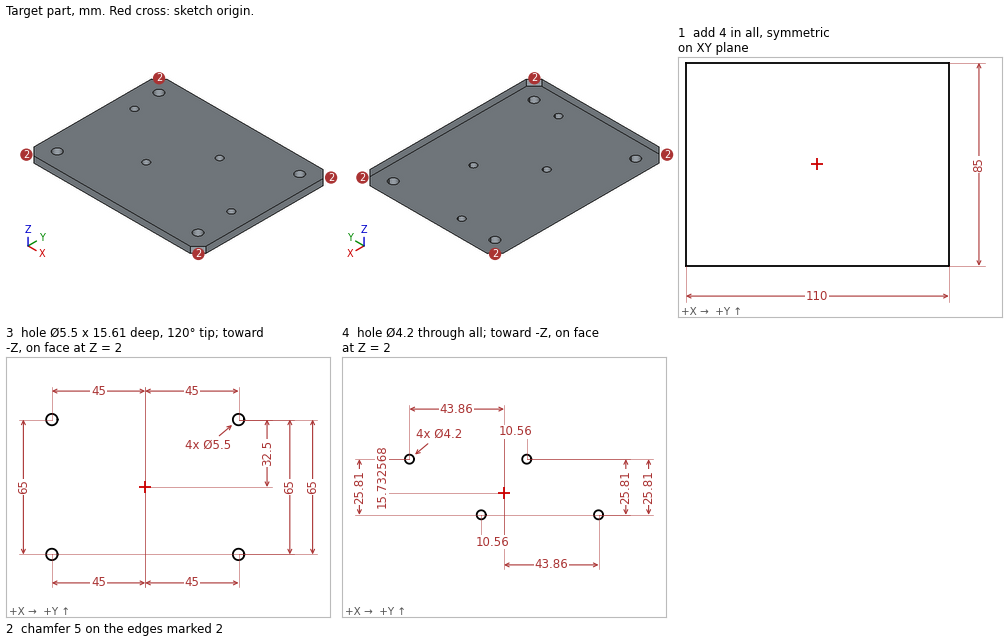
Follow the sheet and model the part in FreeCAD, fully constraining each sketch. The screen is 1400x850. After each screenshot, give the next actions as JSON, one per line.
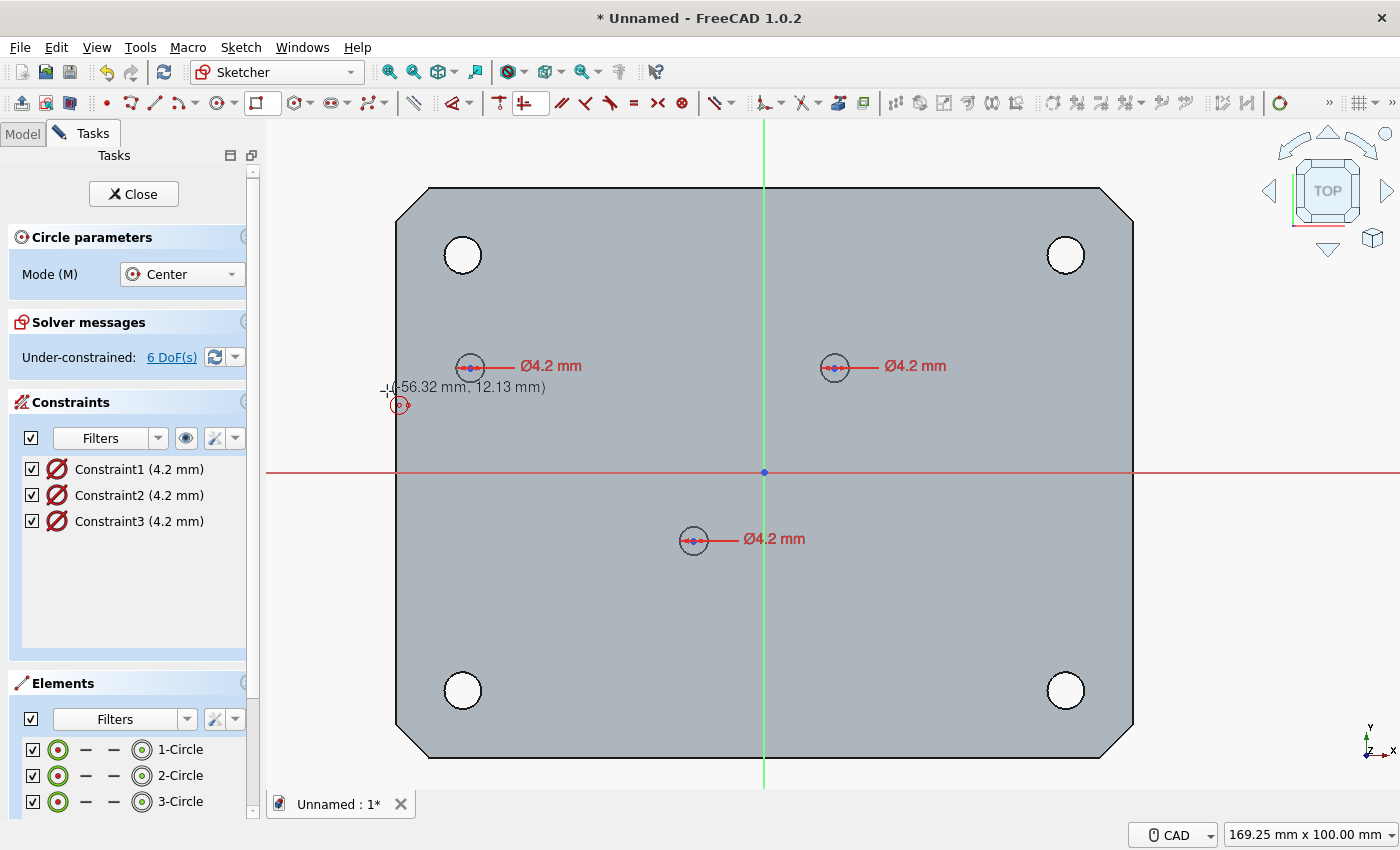
{"action": "scroll", "coordinate": [1058, 540], "scroll_direction": "up", "scroll_amount": 3}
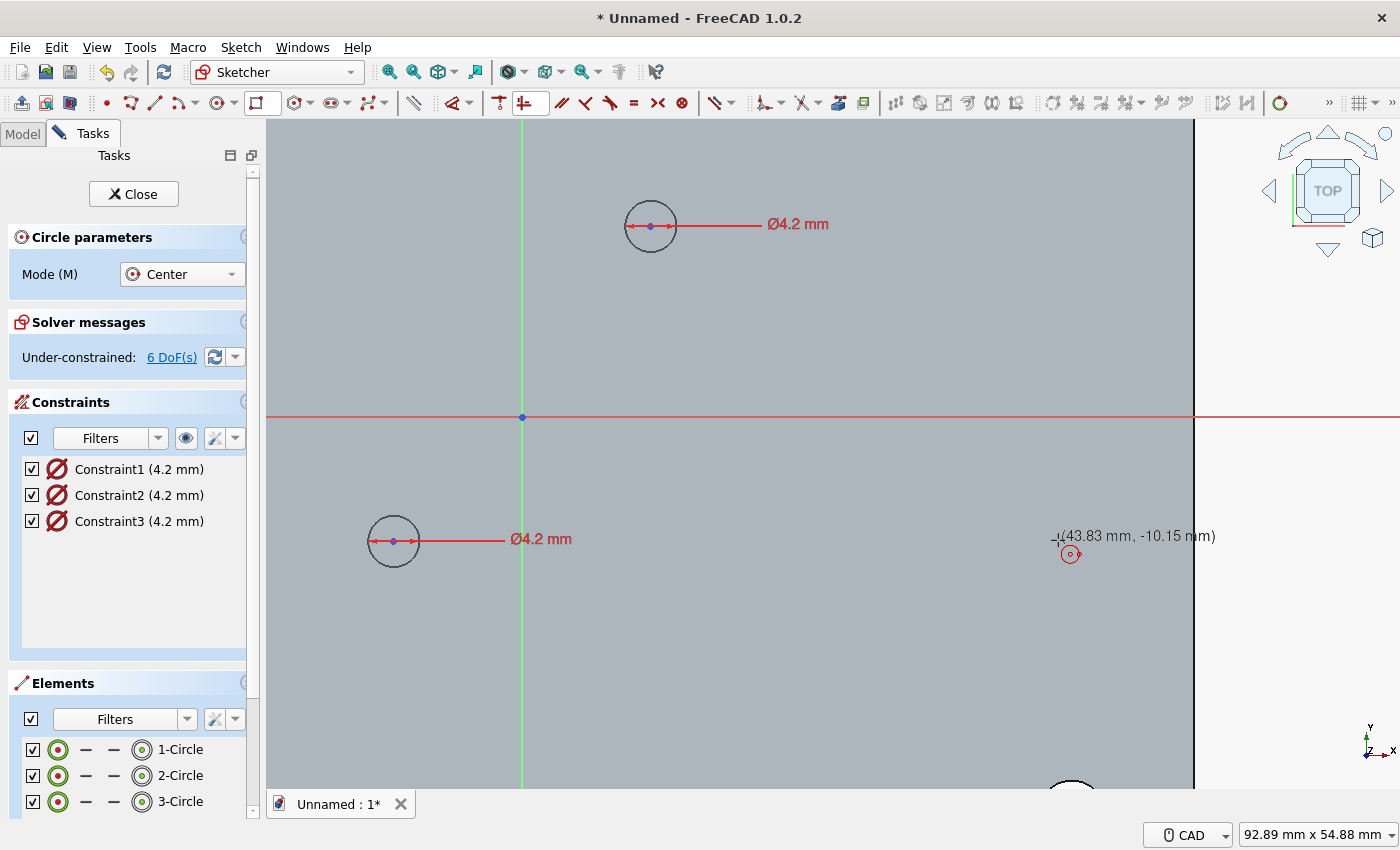
{"action": "left_click", "coordinate": [1058, 540]}
{"action": "mouse_move", "coordinate": [1076, 522]}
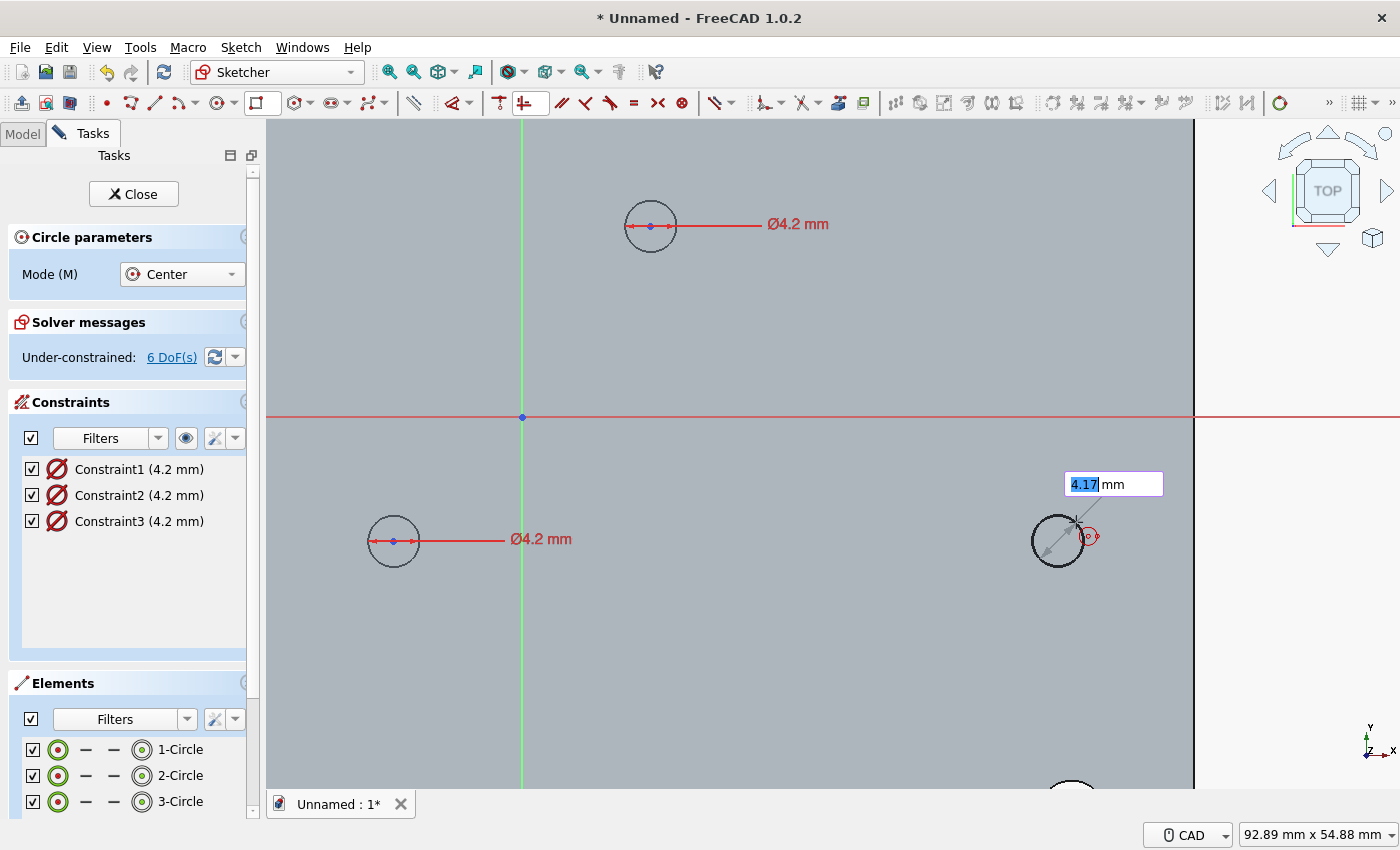
{"action": "type", "text": "4.2"}
{"action": "key", "text": "Return"}
{"action": "key", "text": "Escape"}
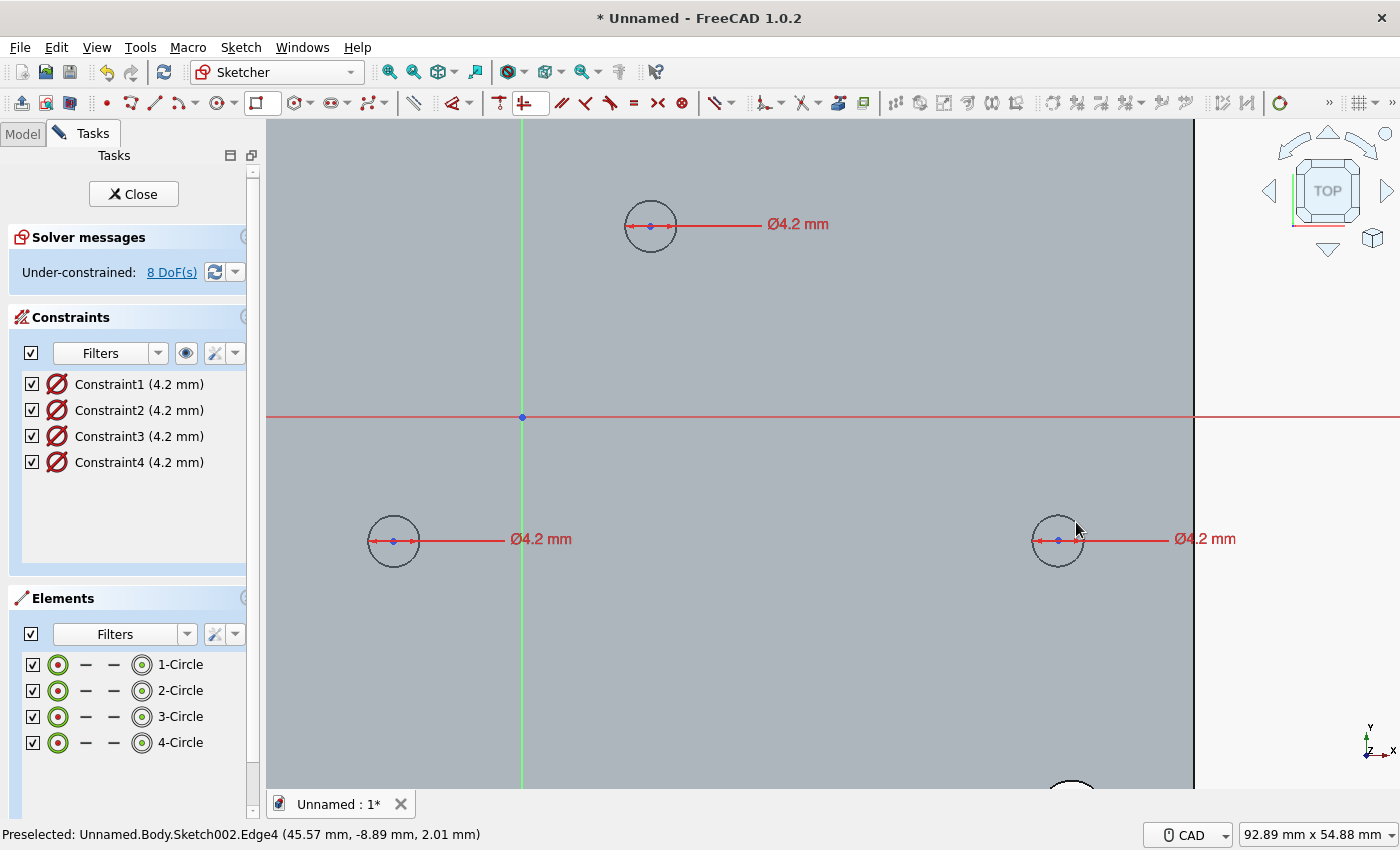
{"action": "key", "text": "d"}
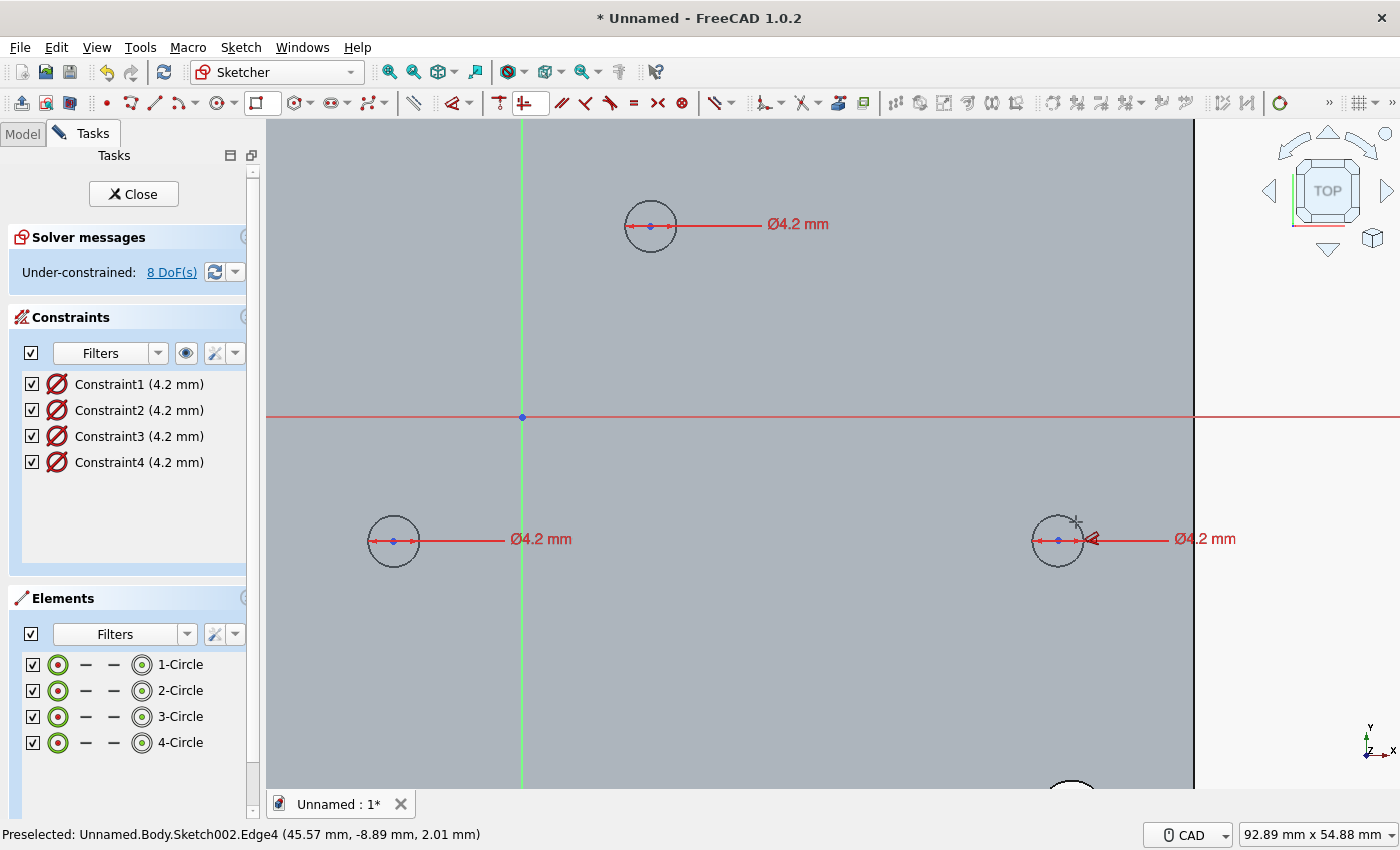
{"action": "scroll", "coordinate": [1059, 541], "scroll_direction": "down", "scroll_amount": 3}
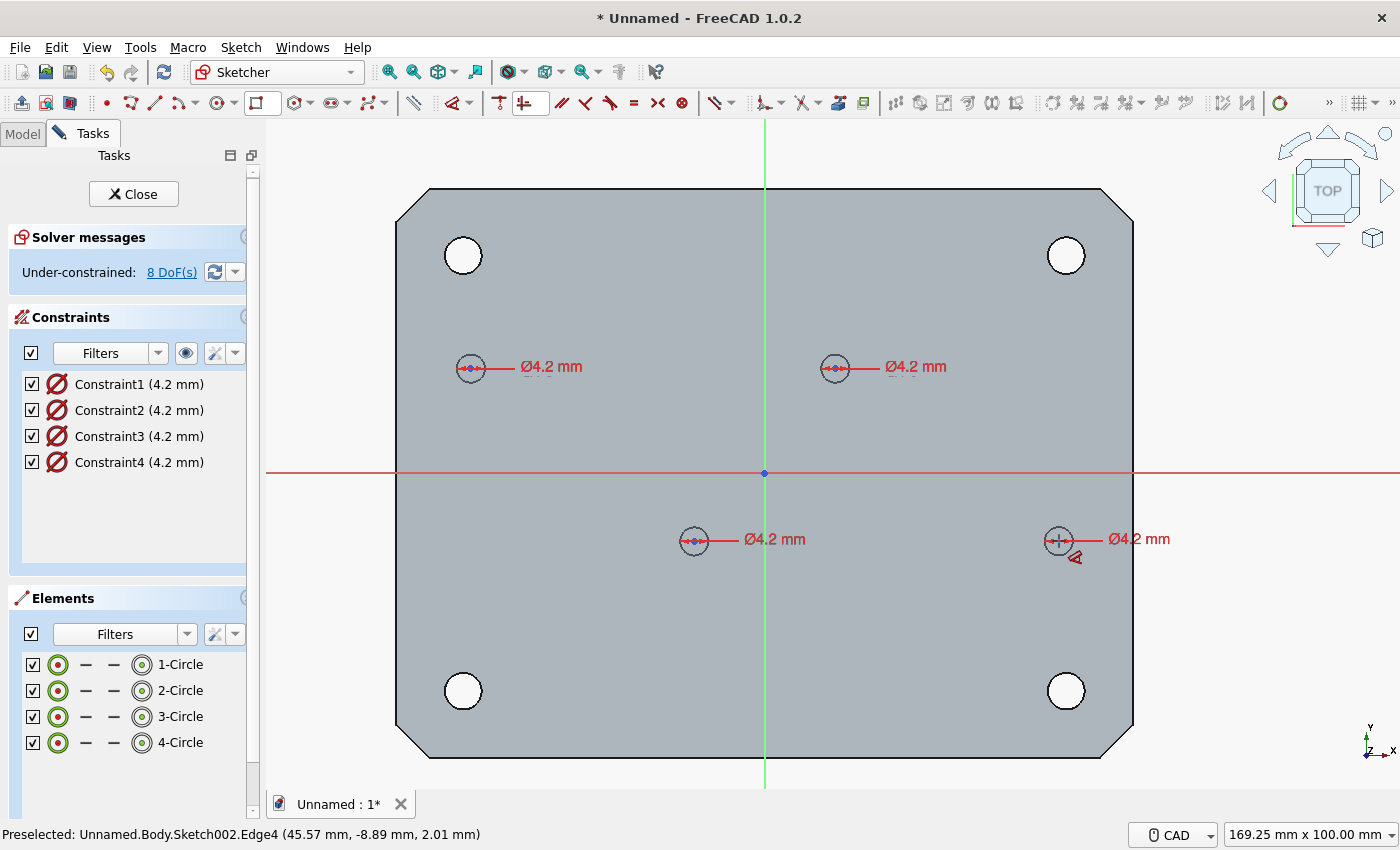
{"action": "left_click", "coordinate": [471, 369]}
{"action": "left_click", "coordinate": [618, 335]}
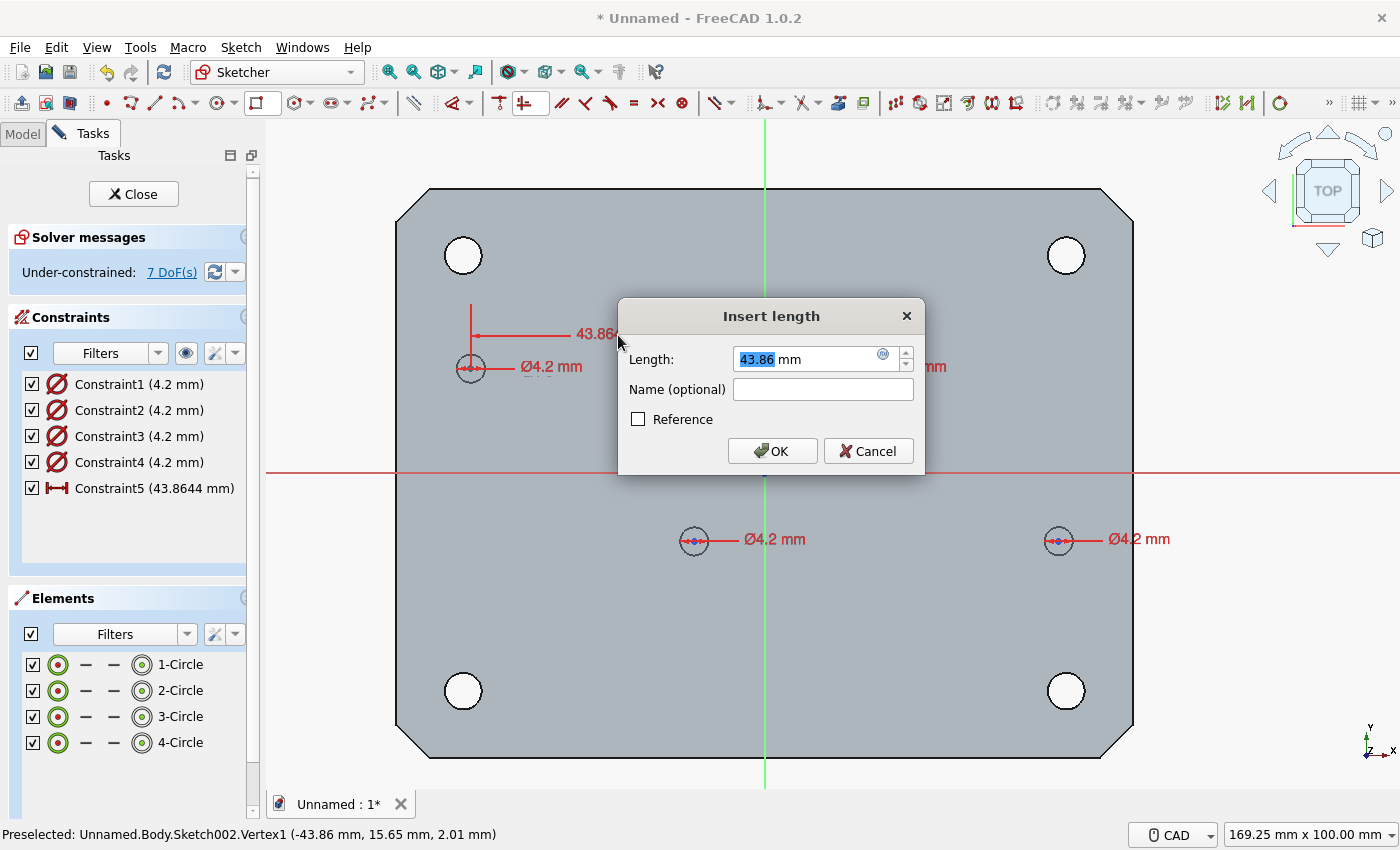
{"action": "type", "text": "43.86"}
{"action": "key", "text": "Return"}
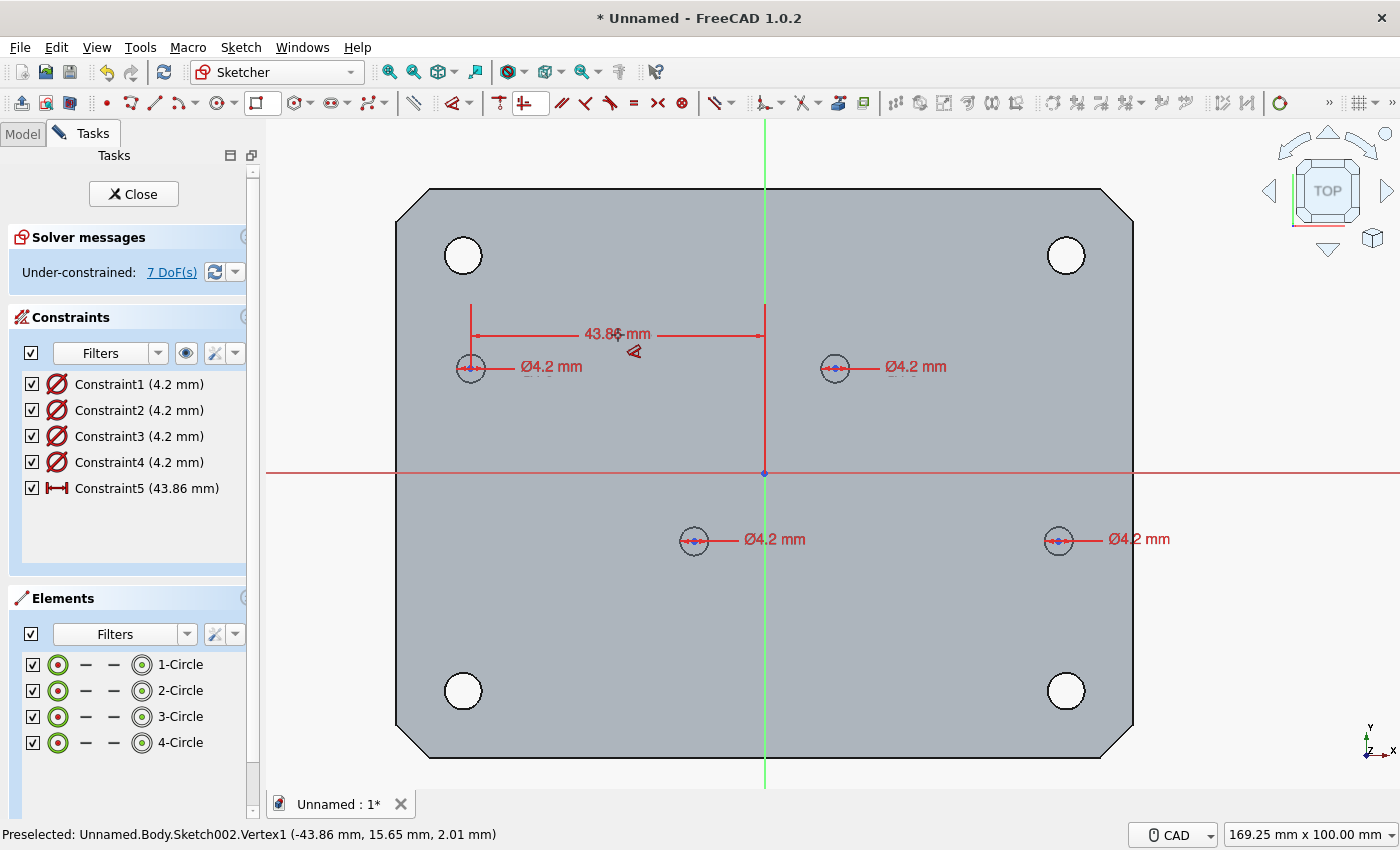
{"action": "left_click", "coordinate": [835, 369]}
{"action": "left_click", "coordinate": [800, 335]}